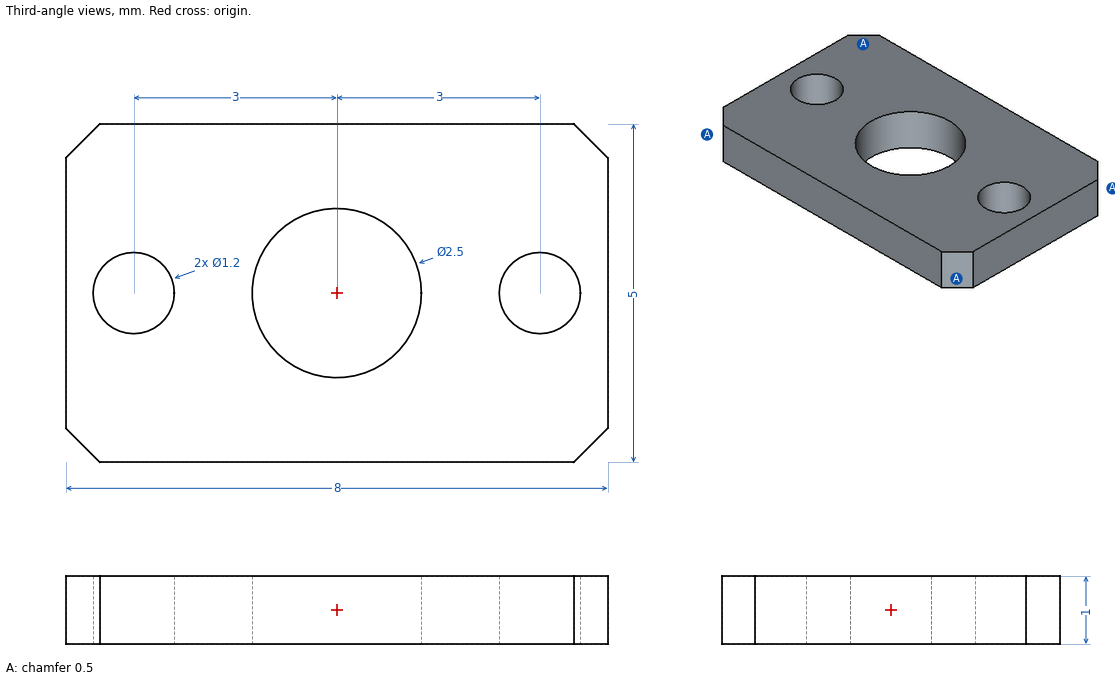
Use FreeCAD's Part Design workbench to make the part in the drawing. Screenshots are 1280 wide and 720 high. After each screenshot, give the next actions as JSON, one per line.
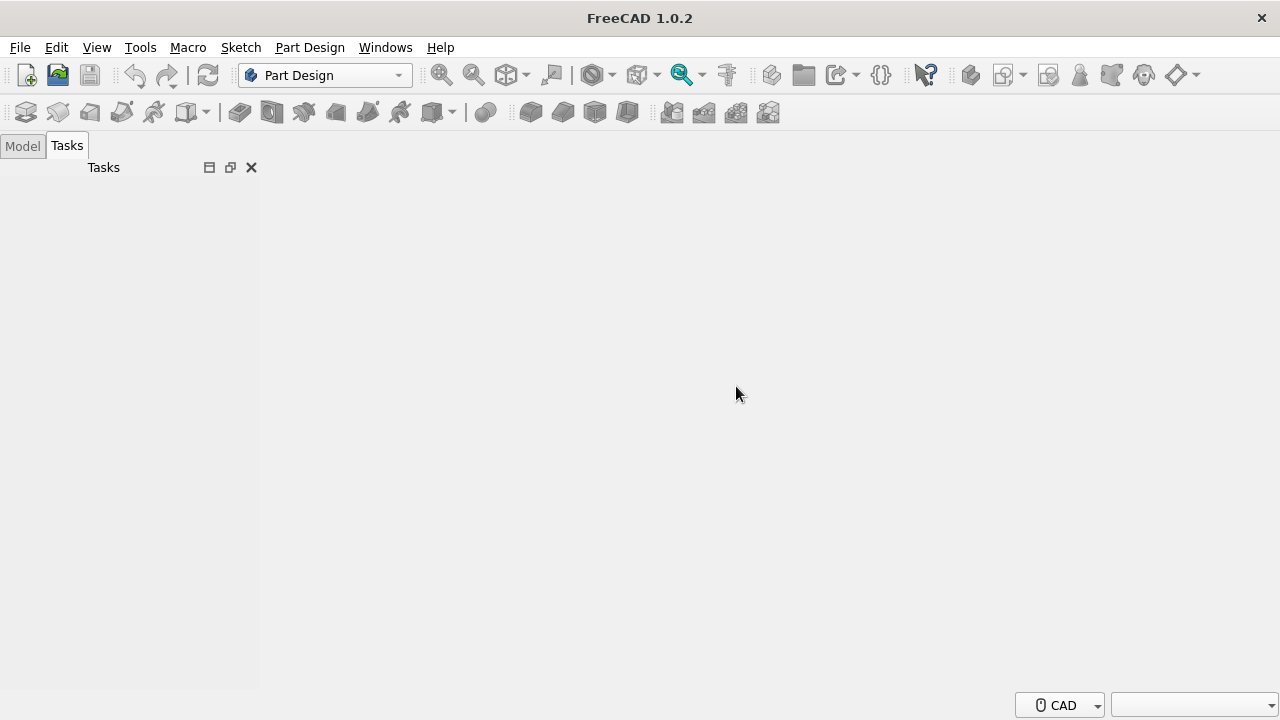
{"action": "left_click", "coordinate": [26, 76]}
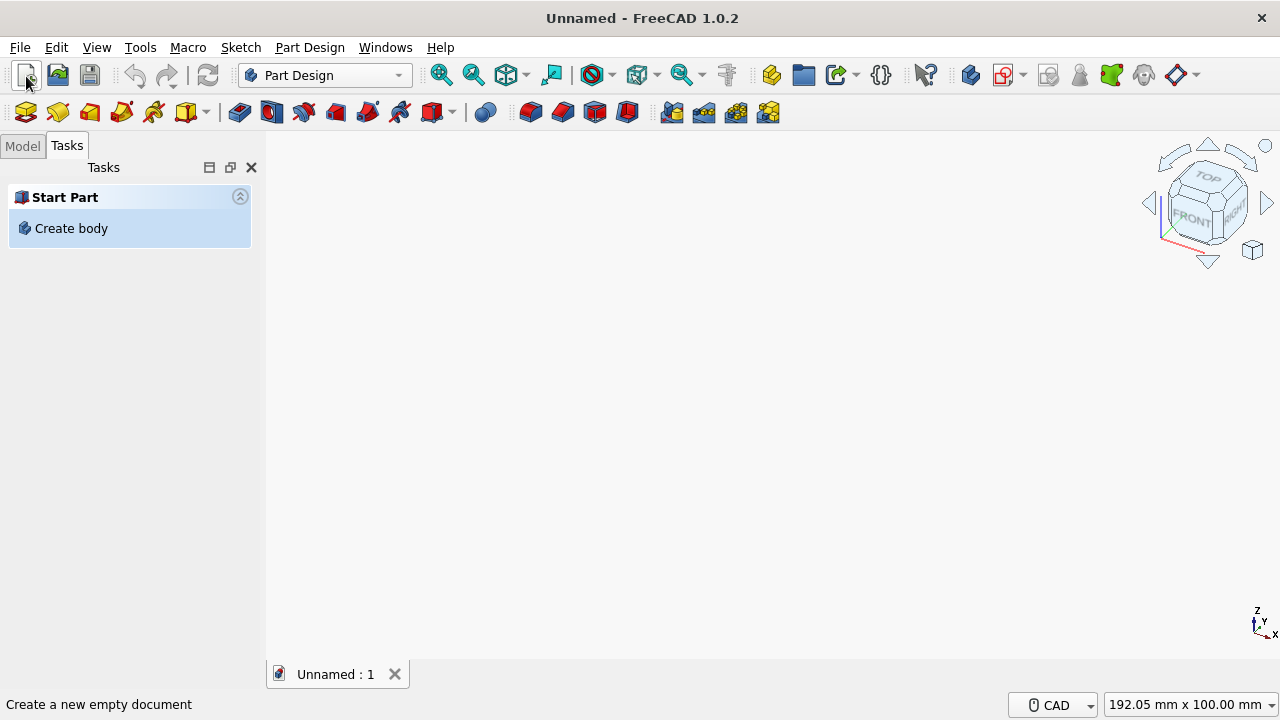
{"action": "left_click", "coordinate": [1004, 76]}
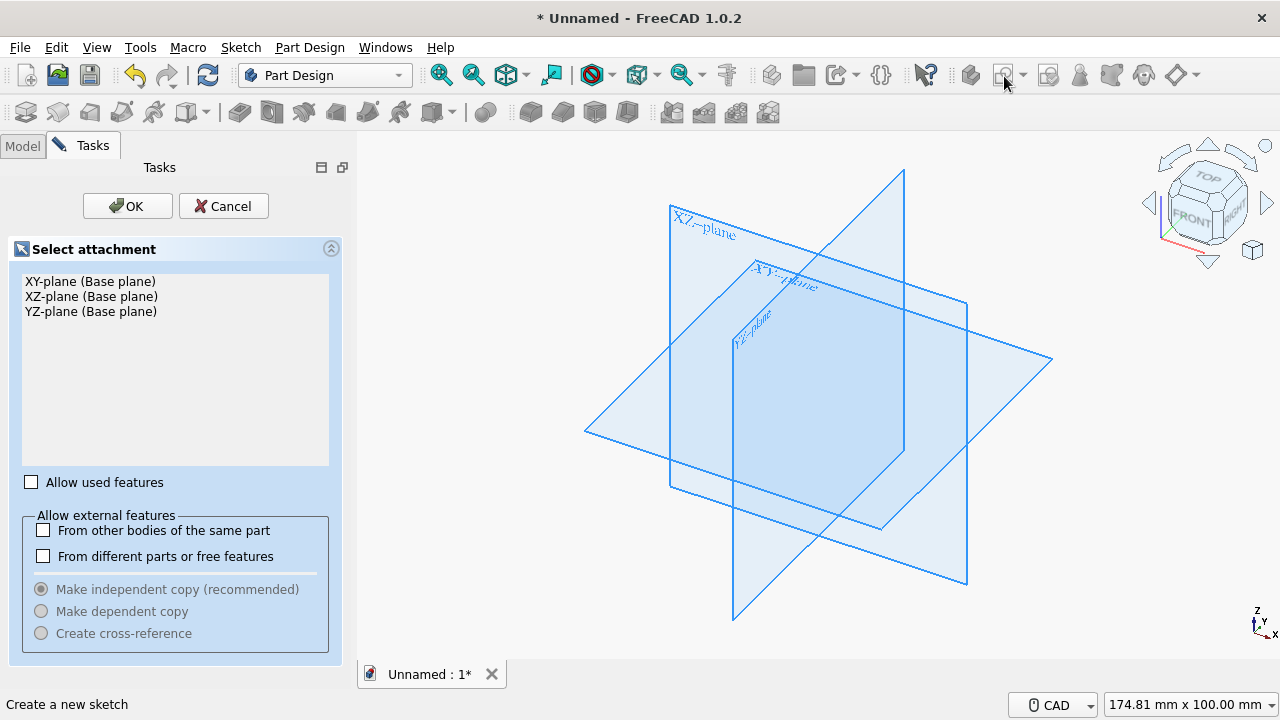
{"action": "left_click", "coordinate": [82, 282]}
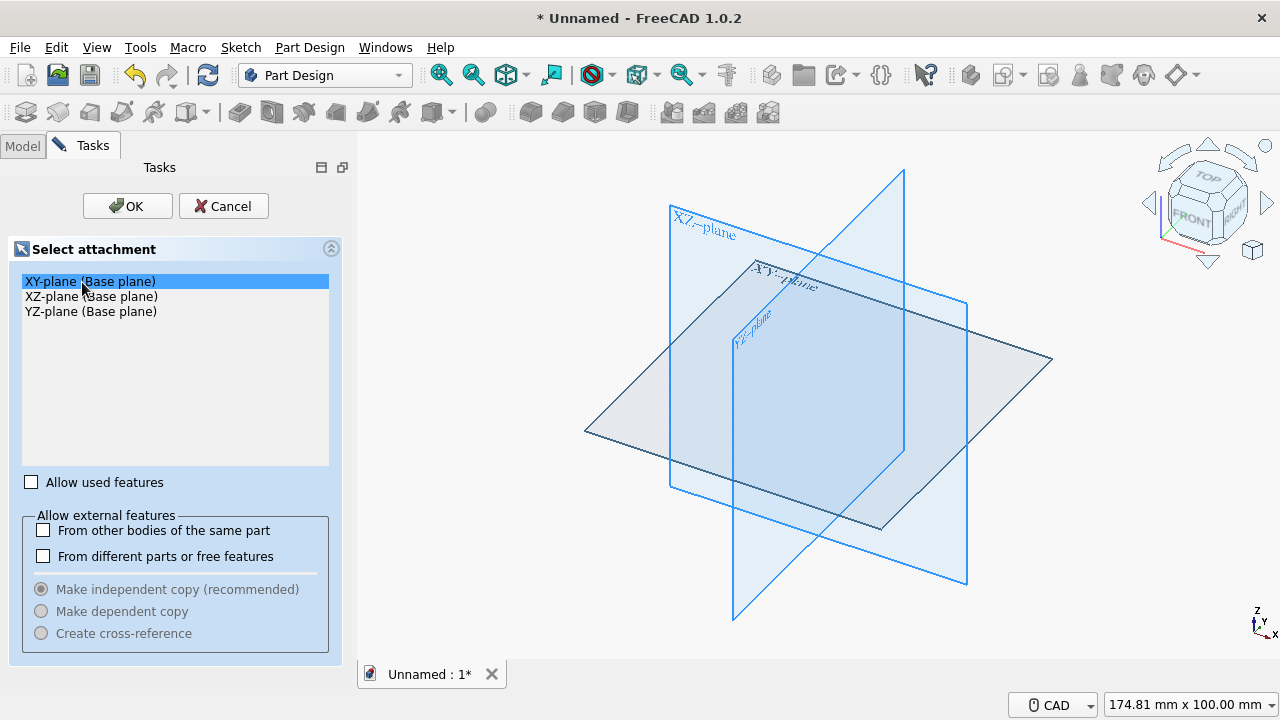
{"action": "left_click", "coordinate": [128, 206]}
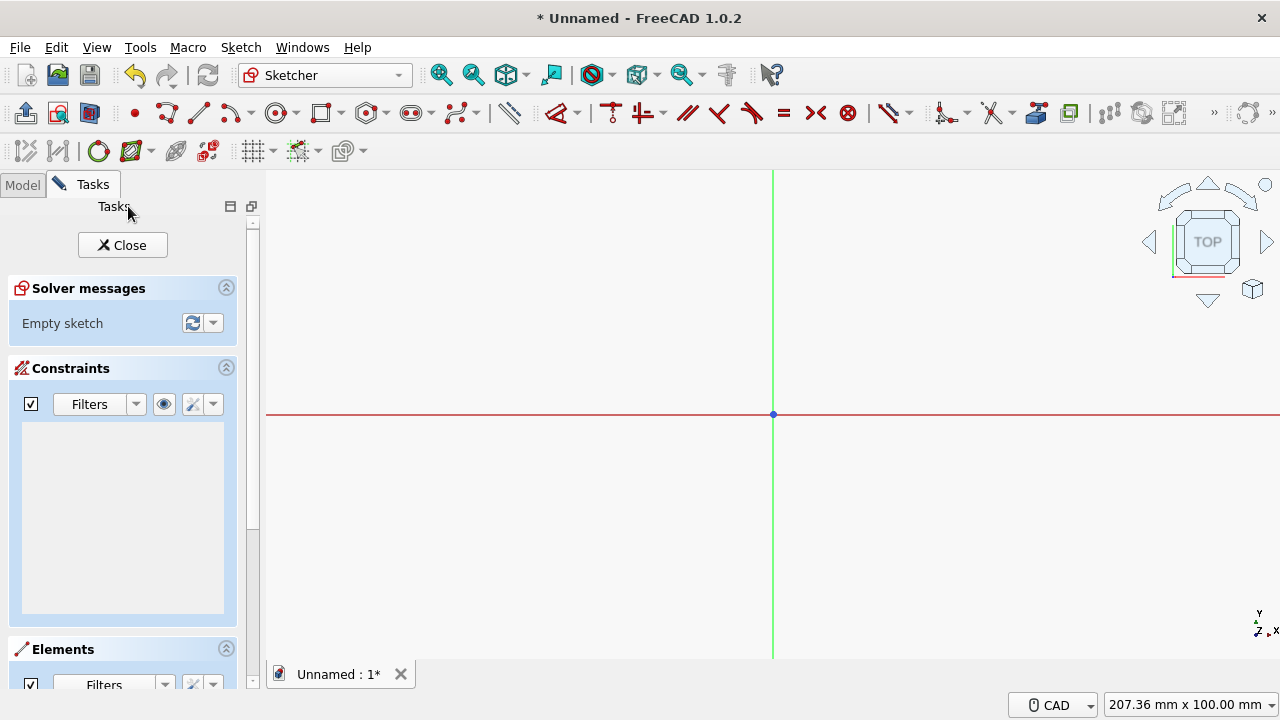
{"action": "scroll", "coordinate": [778, 415], "scroll_direction": "up", "scroll_amount": 13}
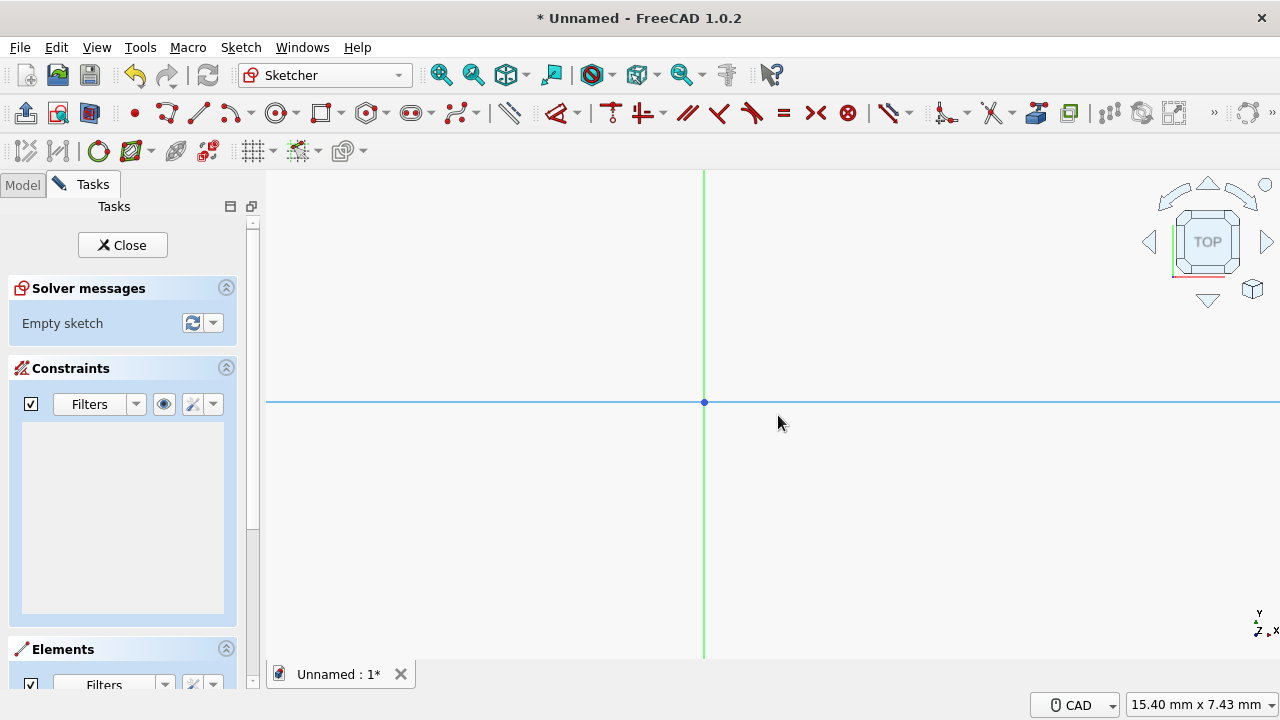
{"action": "key", "text": "g v"}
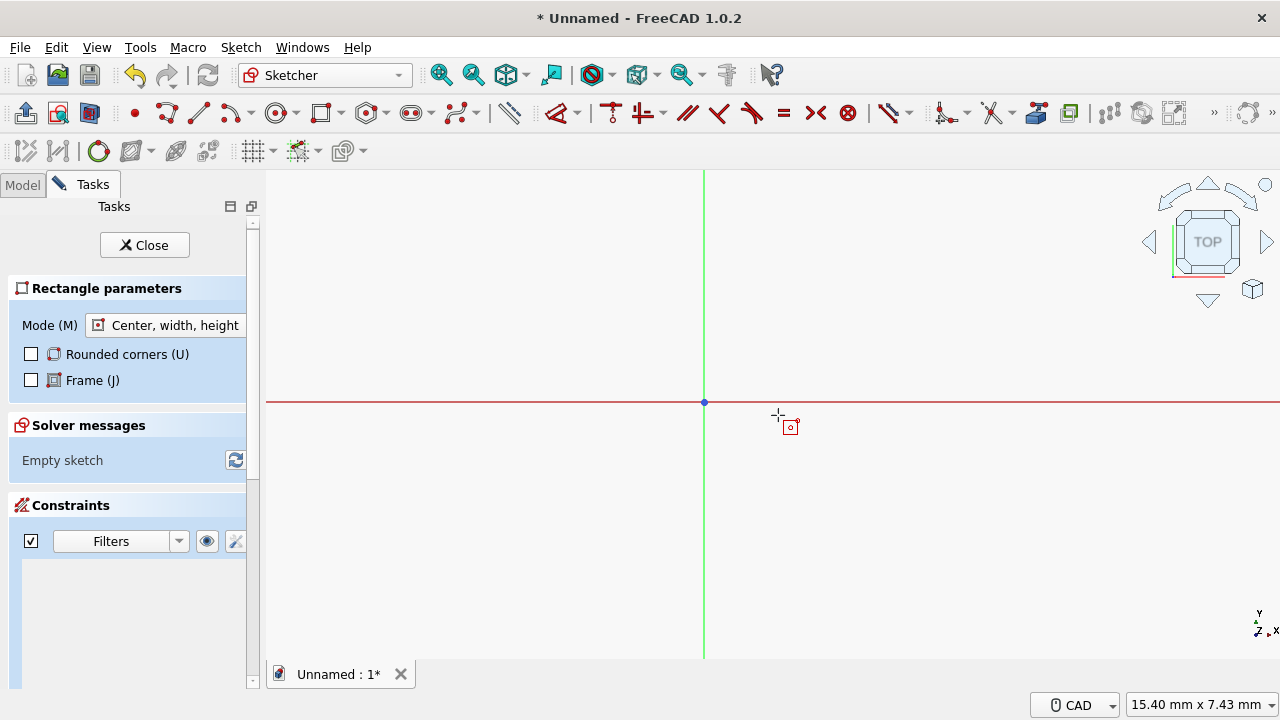
{"action": "left_click", "coordinate": [704, 402]}
{"action": "left_click", "coordinate": [968, 237]}
{"action": "key", "text": "Escape"}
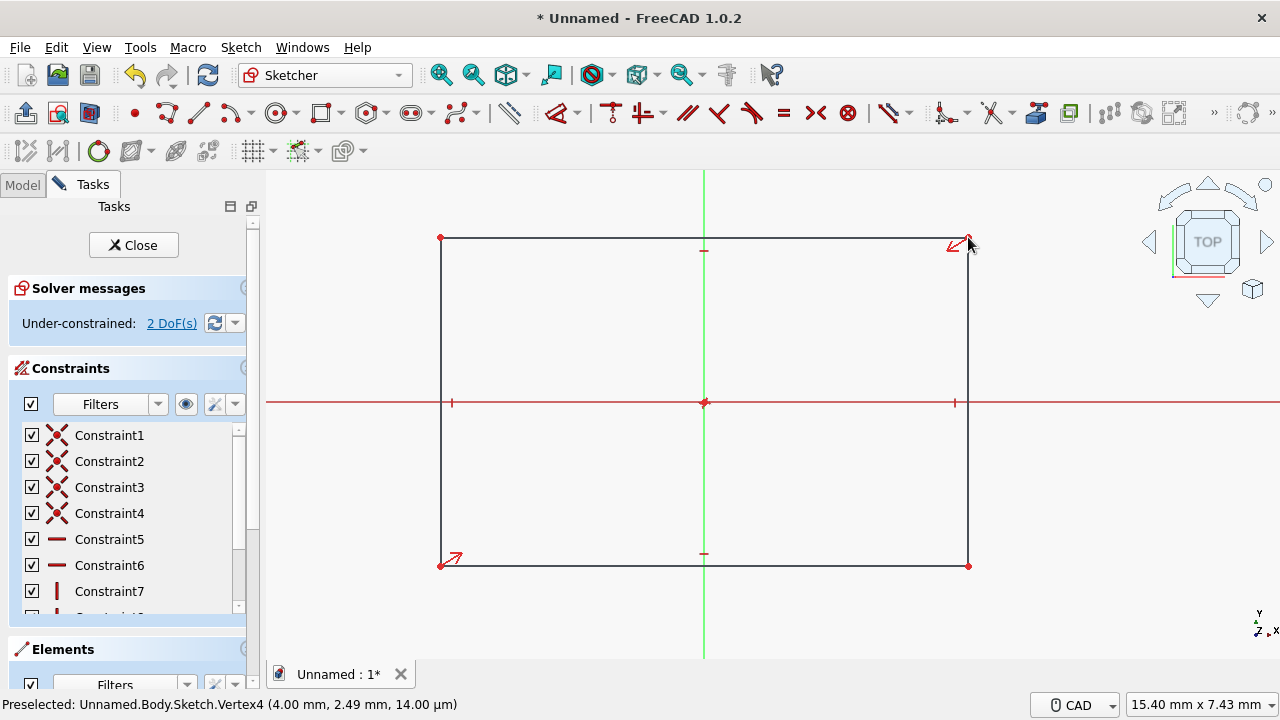
{"action": "left_click", "coordinate": [556, 114]}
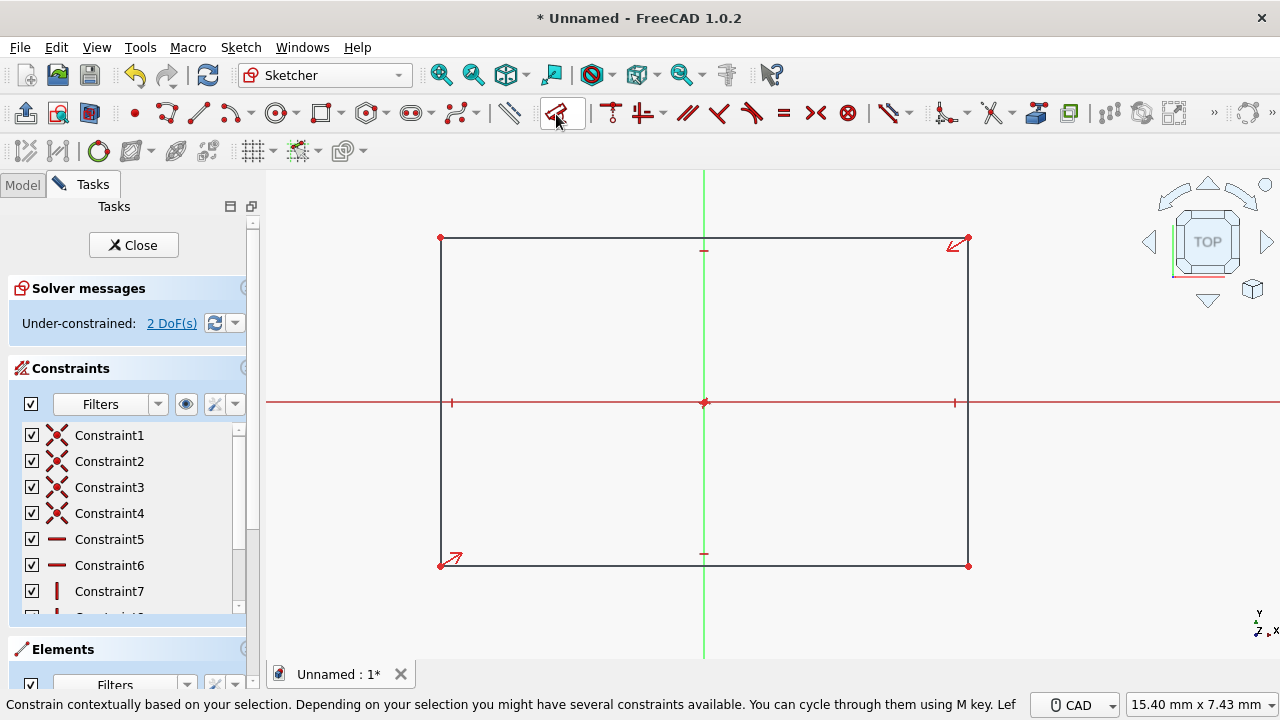
{"action": "left_click", "coordinate": [599, 566]}
{"action": "left_click", "coordinate": [583, 600]}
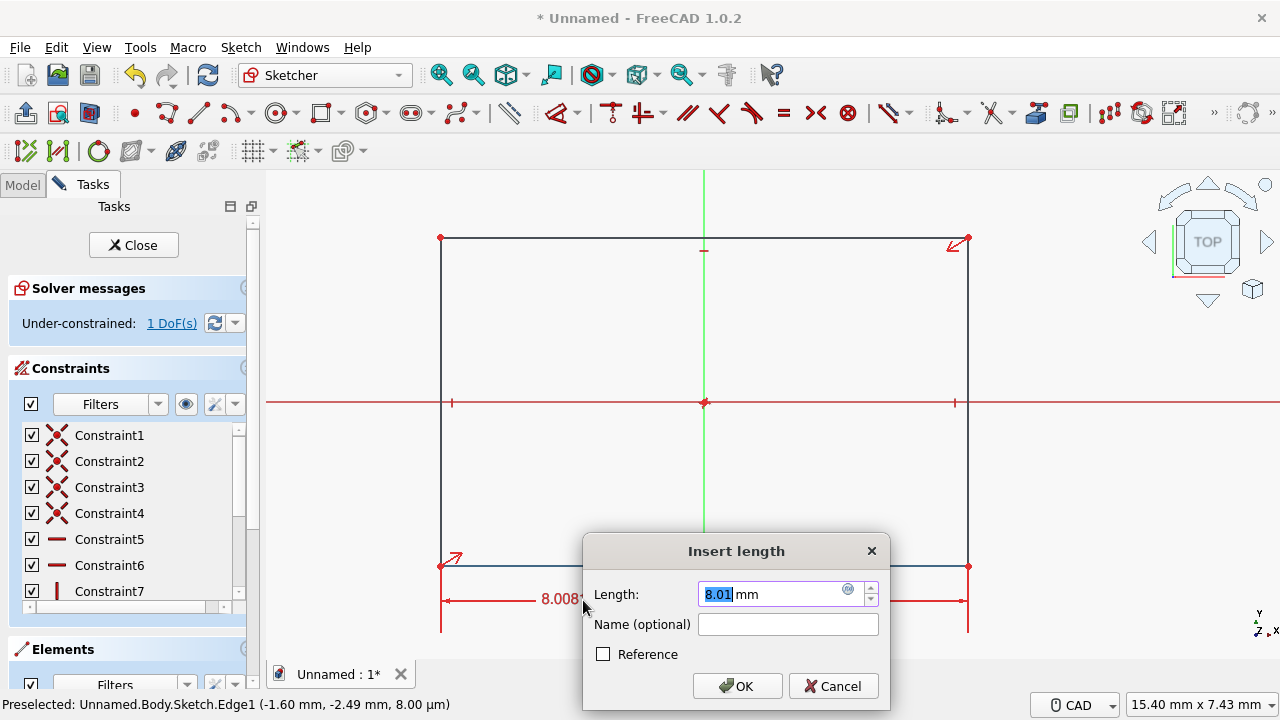
{"action": "type", "text": "8"}
{"action": "key", "text": "Return"}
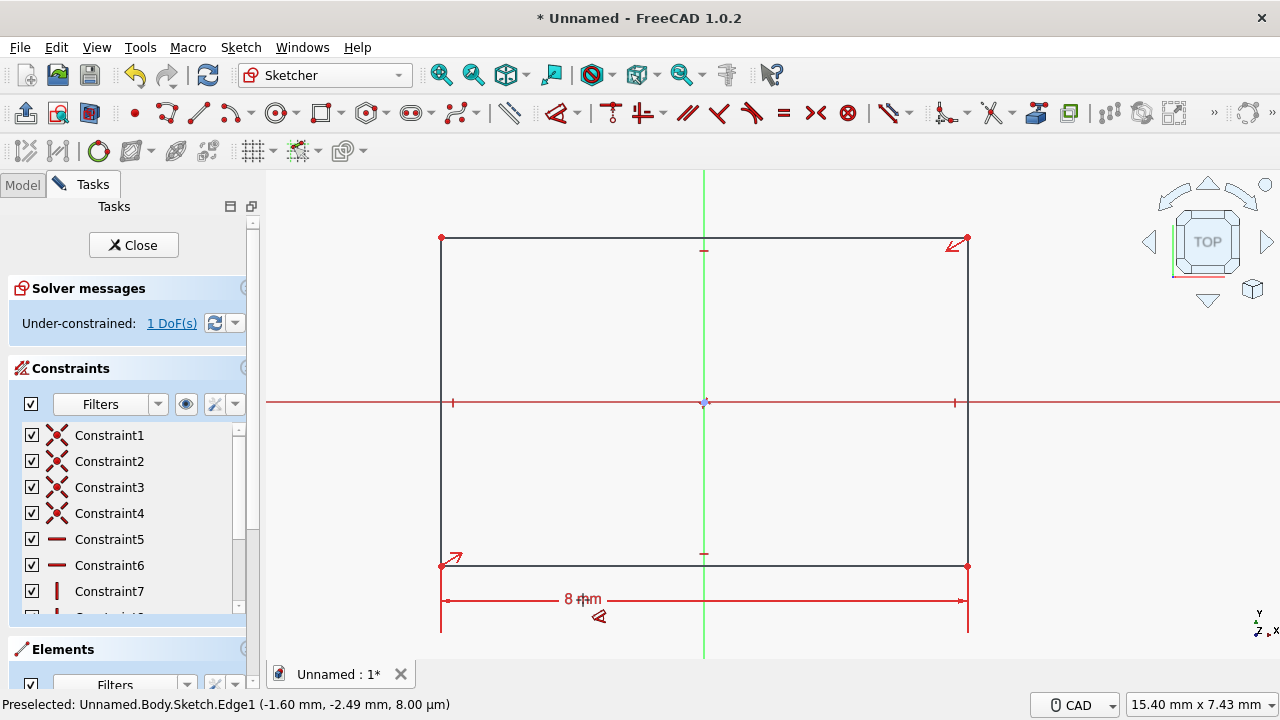
{"action": "left_click", "coordinate": [968, 468]}
{"action": "left_click", "coordinate": [1002, 327]}